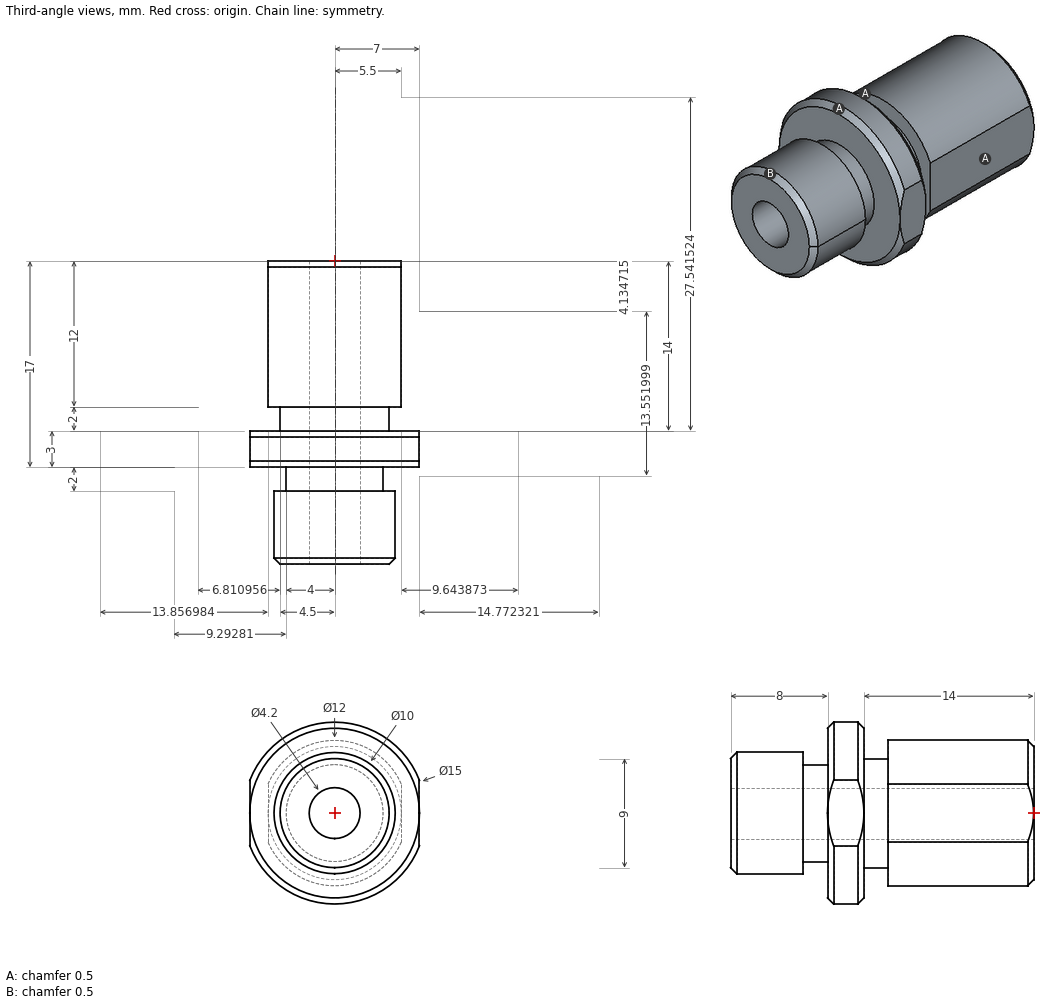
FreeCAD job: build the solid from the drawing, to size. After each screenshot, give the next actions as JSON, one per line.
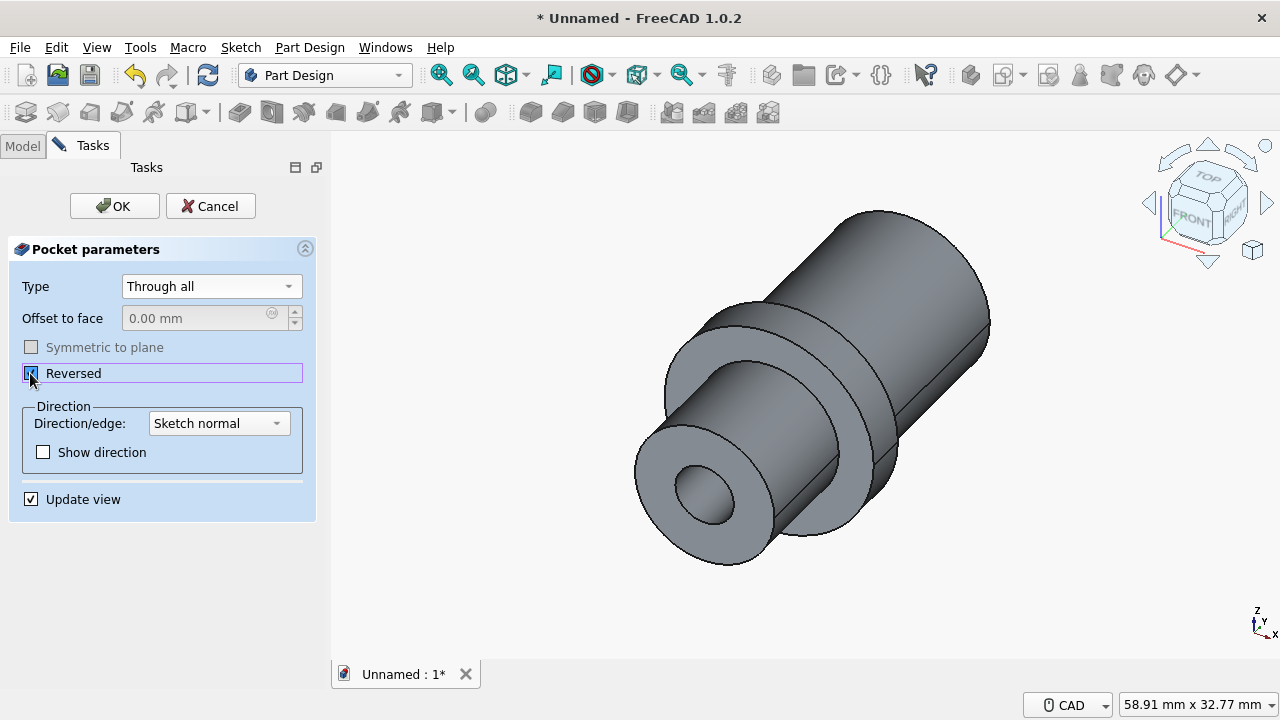
{"action": "left_click", "coordinate": [115, 206]}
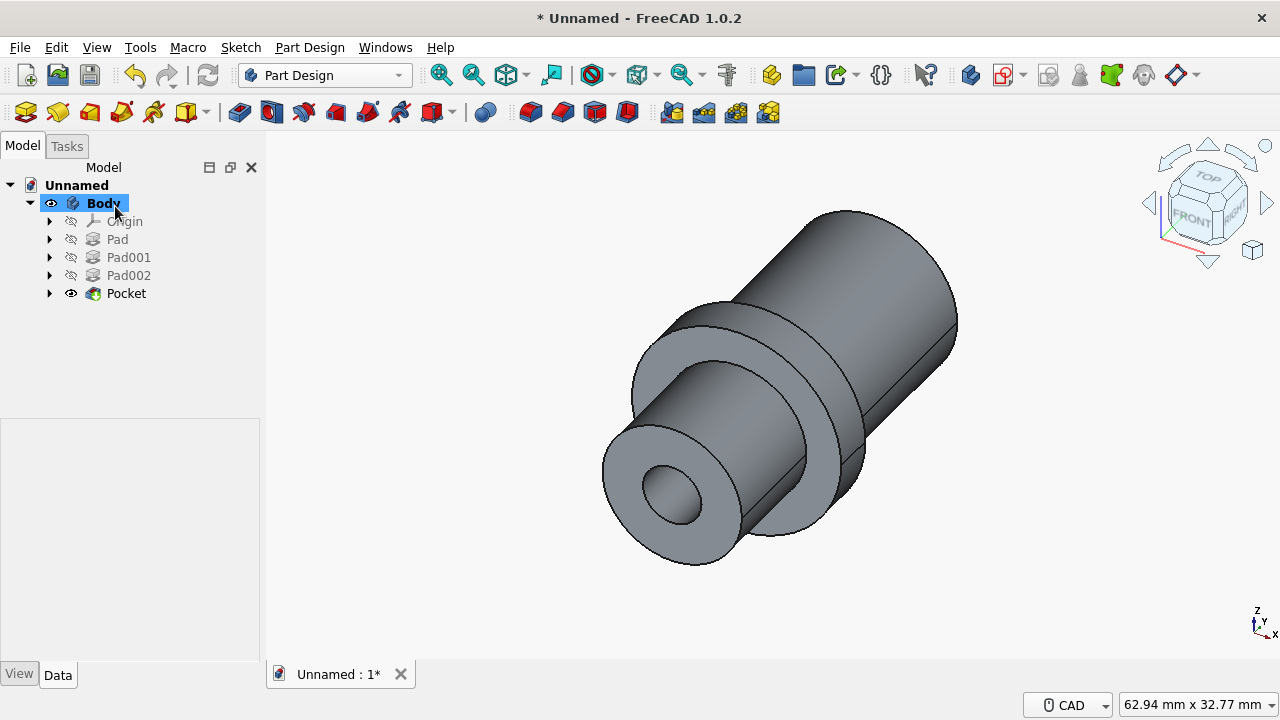
{"action": "left_click", "coordinate": [652, 344]}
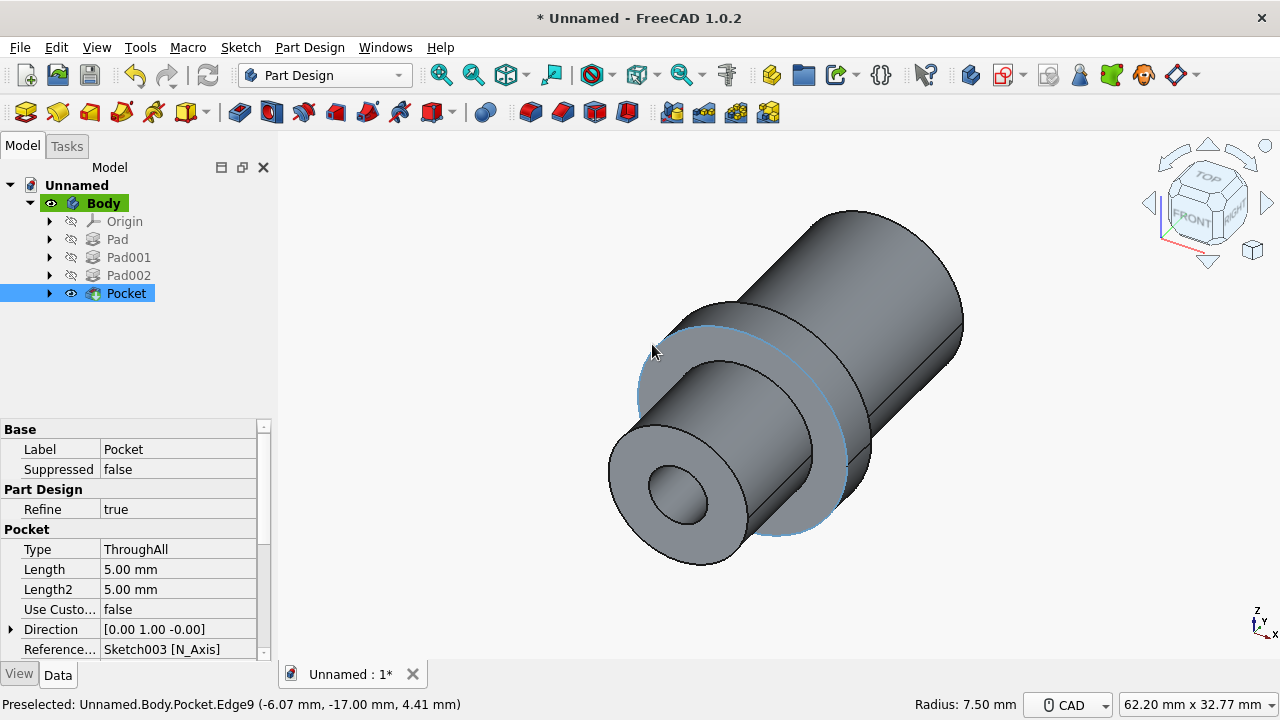
{"action": "key", "text": "0"}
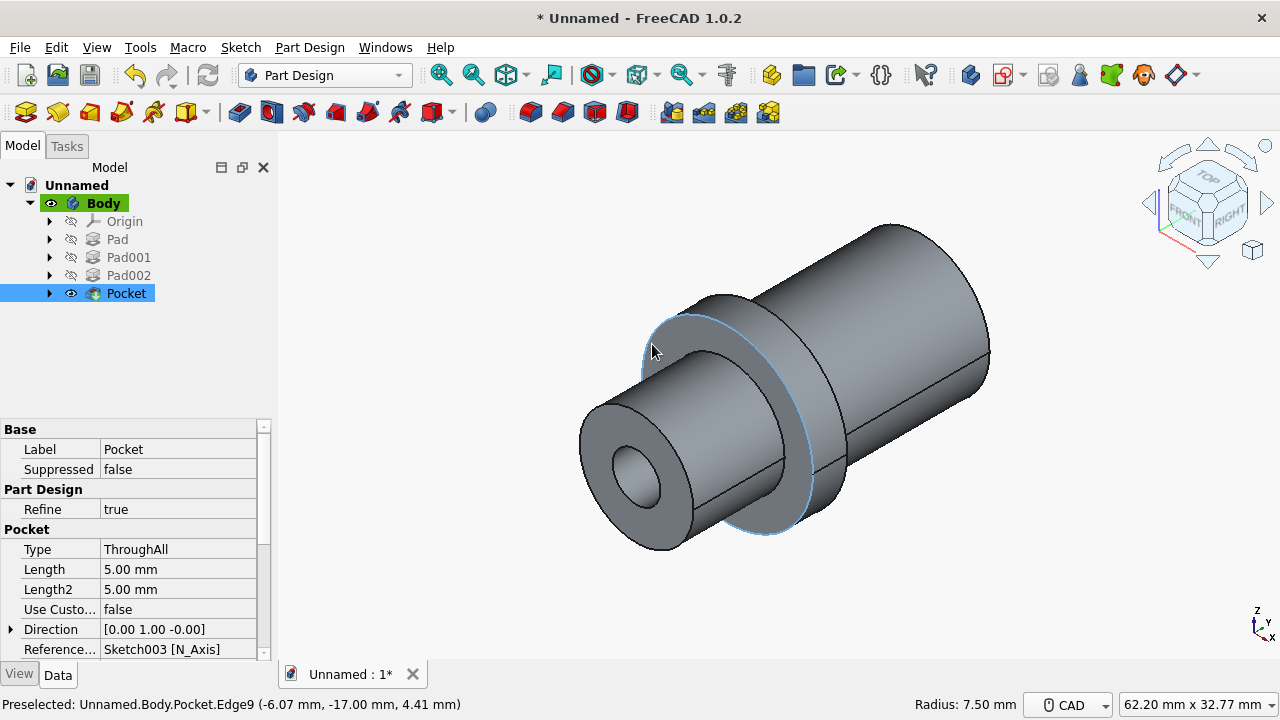
{"action": "key", "text": "2"}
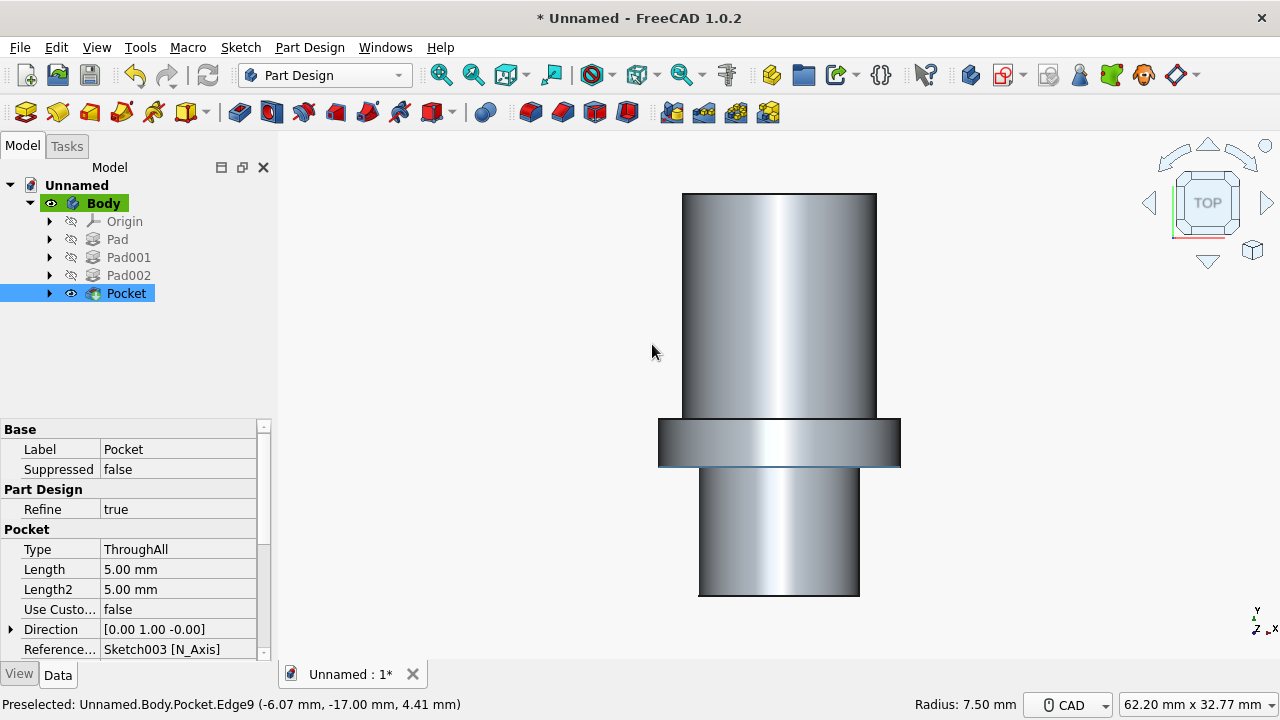
{"action": "left_click", "coordinate": [701, 193], "text": "ctrl"}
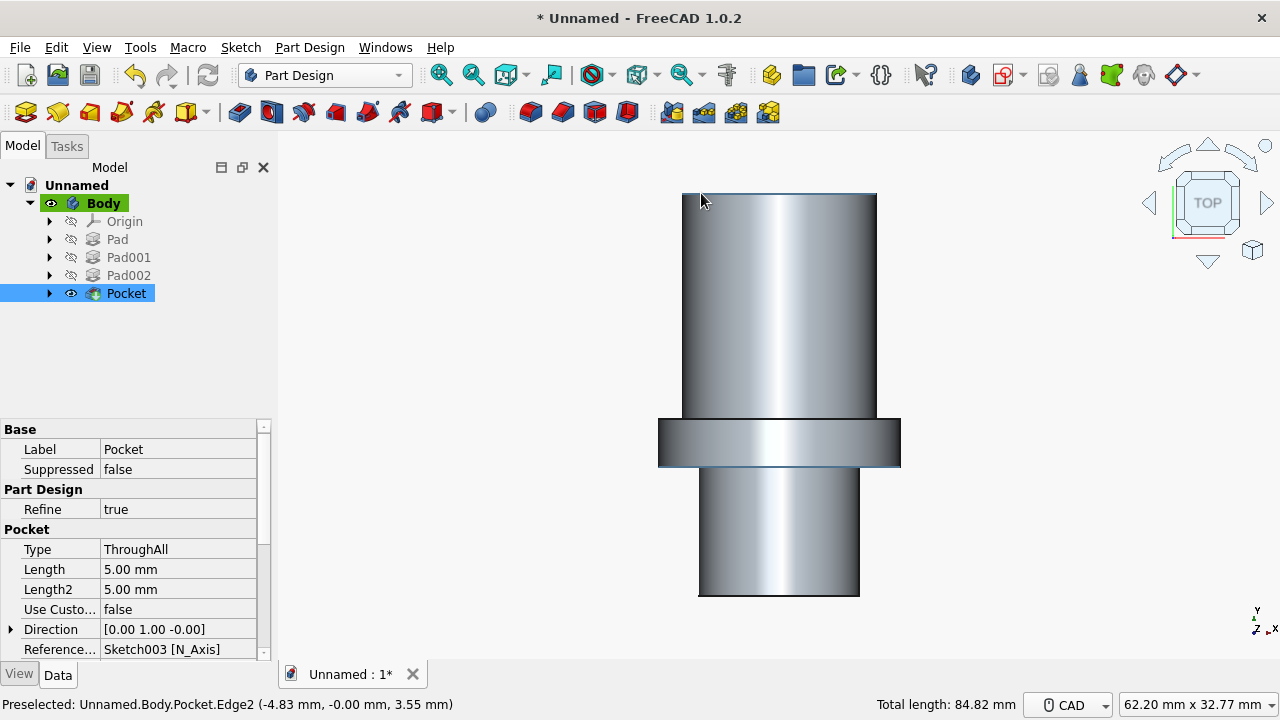
{"action": "left_click", "coordinate": [681, 418], "text": "ctrl"}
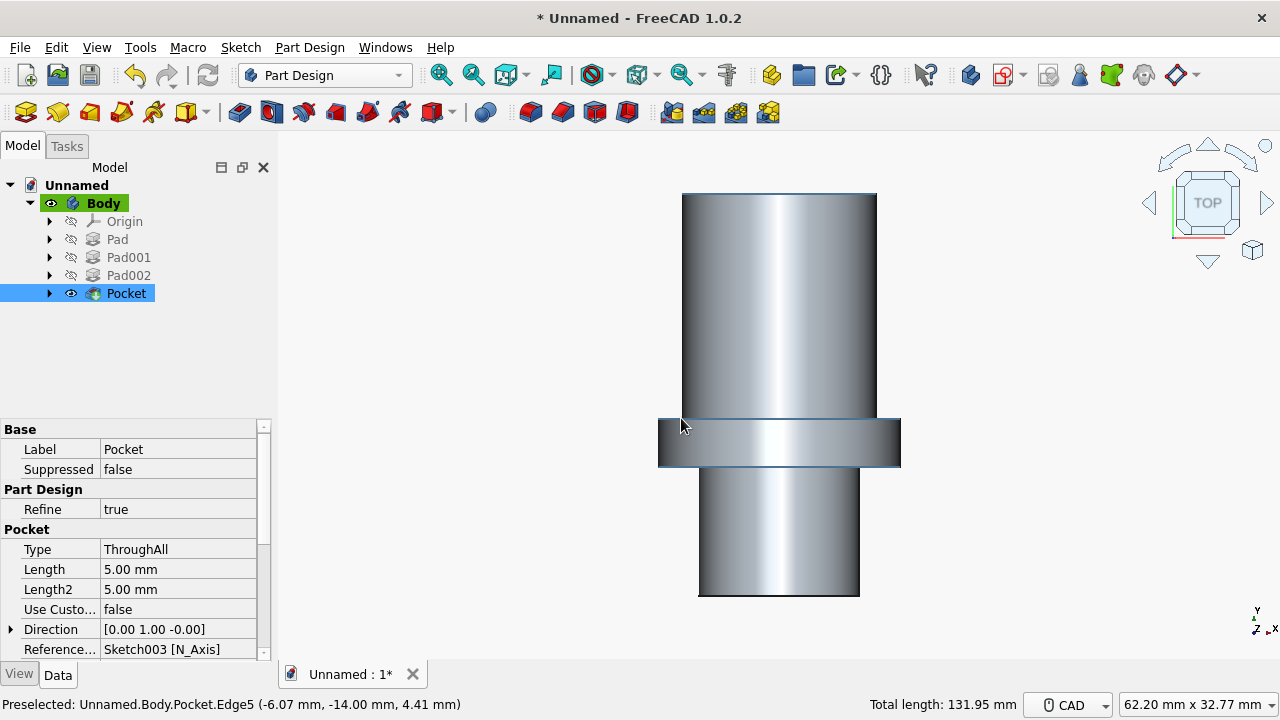
{"action": "left_click", "coordinate": [564, 112]}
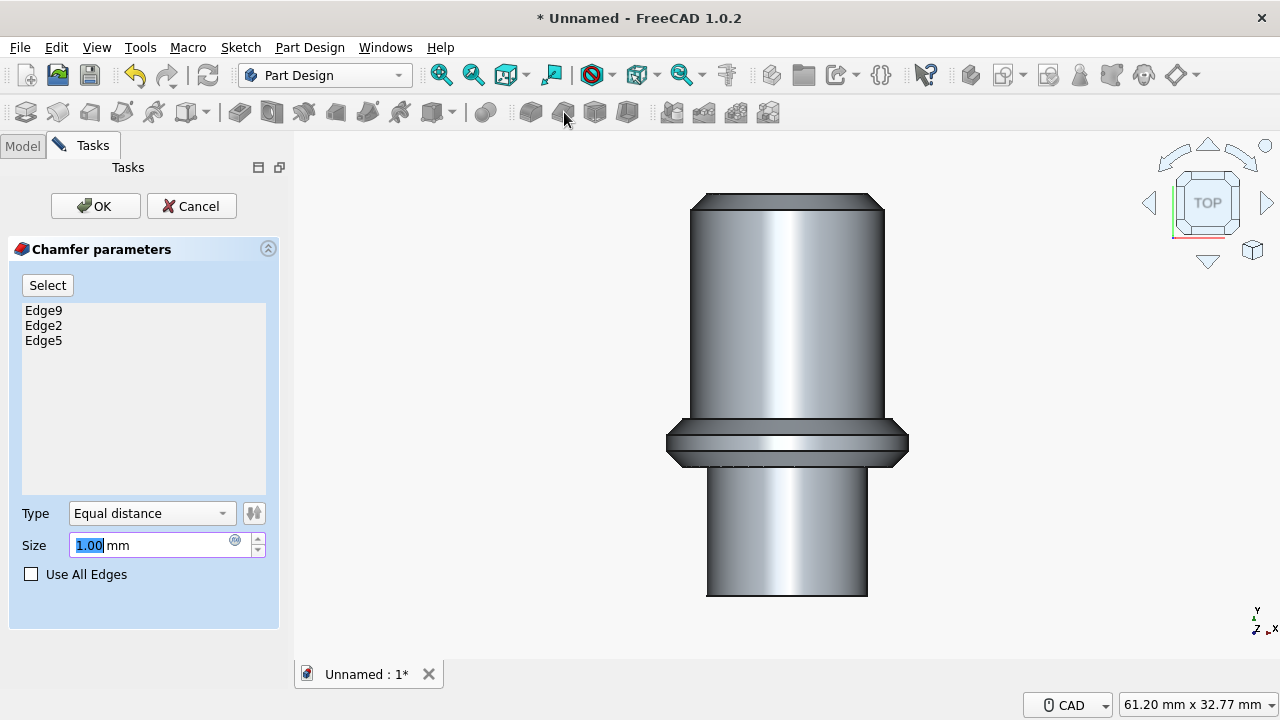
{"action": "type", "text": "0.5"}
{"action": "key", "text": "Tab"}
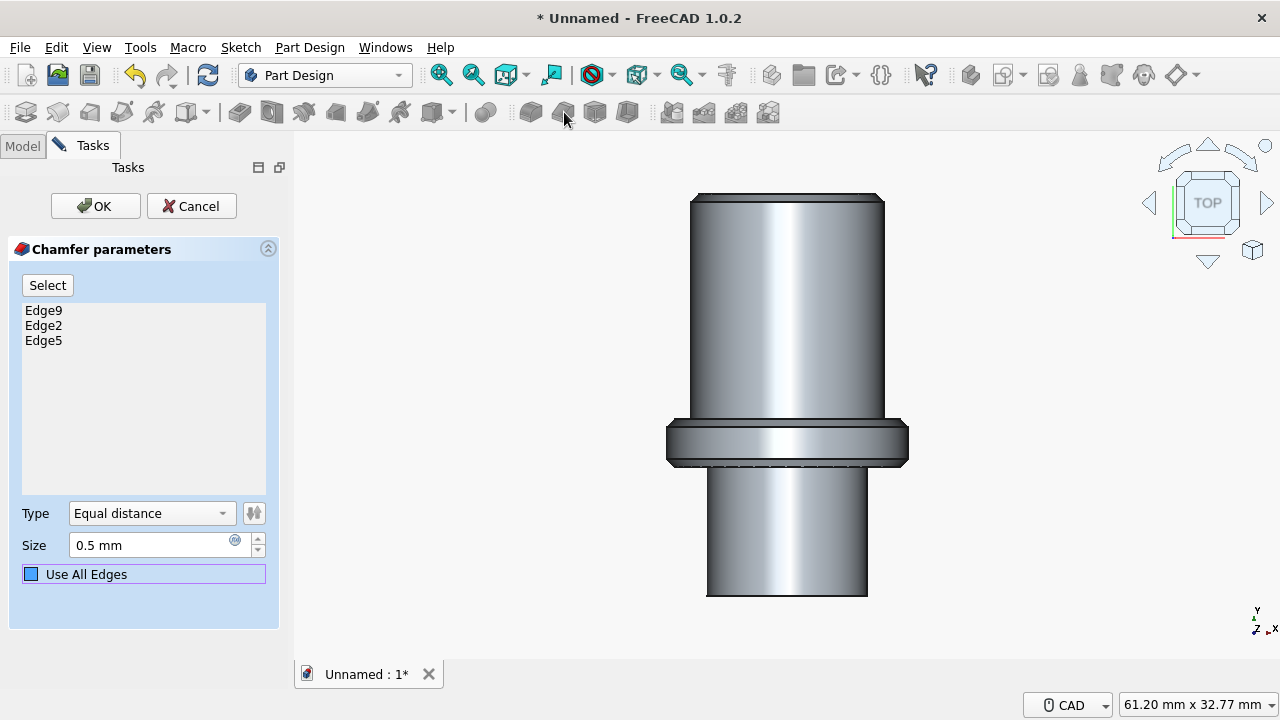
{"action": "left_click", "coordinate": [96, 206]}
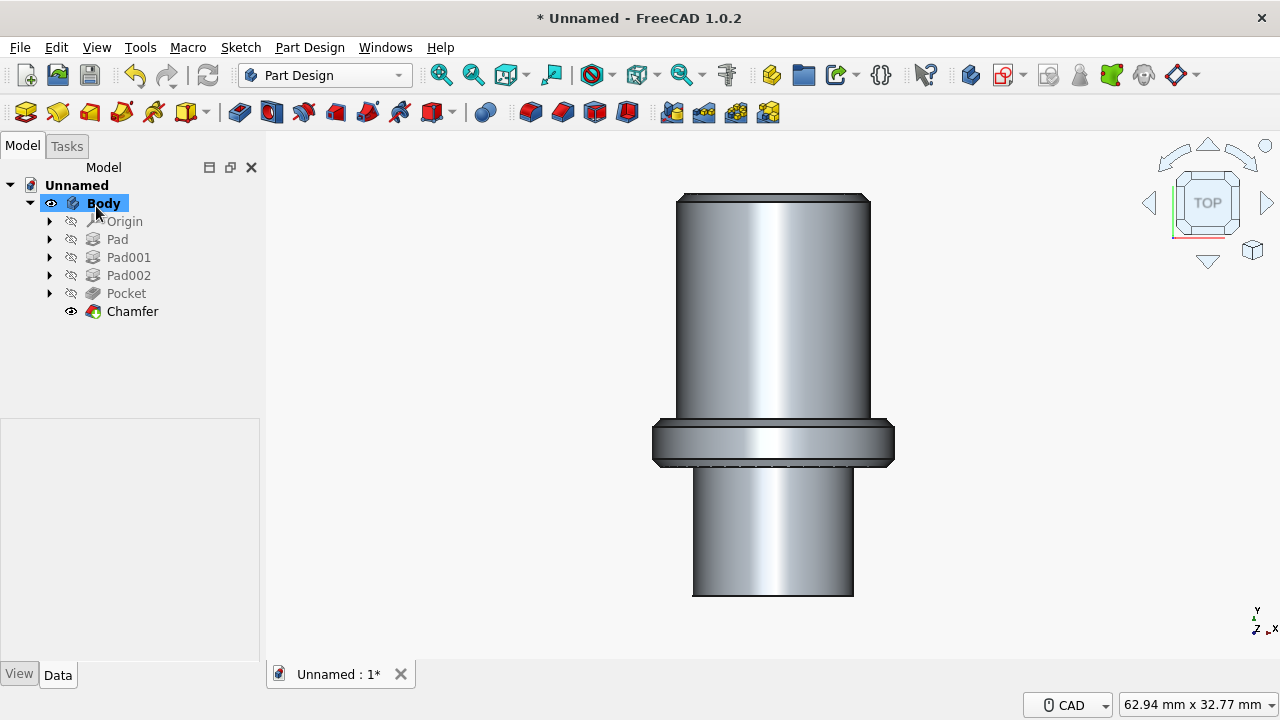
{"action": "left_click", "coordinate": [1004, 76]}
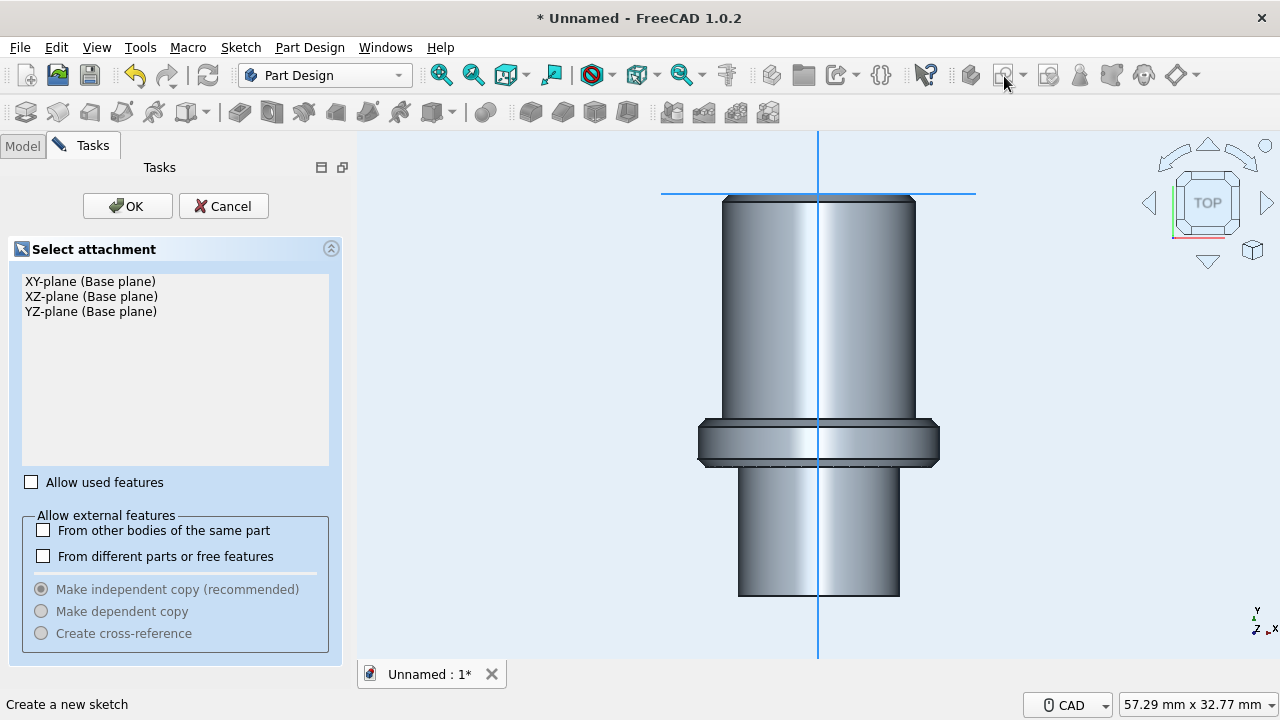
{"action": "left_click", "coordinate": [82, 282]}